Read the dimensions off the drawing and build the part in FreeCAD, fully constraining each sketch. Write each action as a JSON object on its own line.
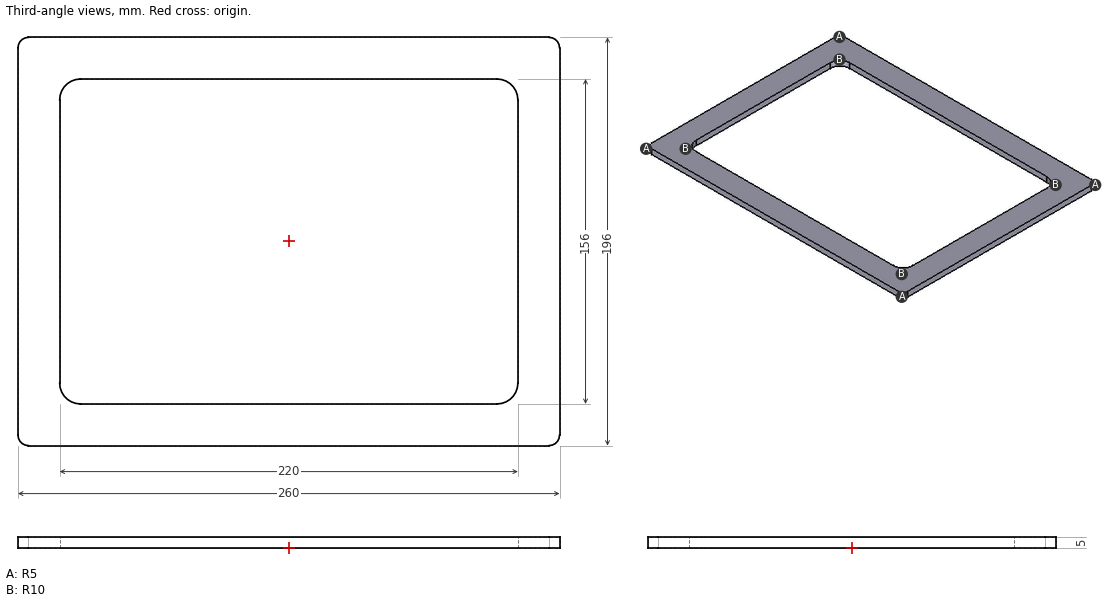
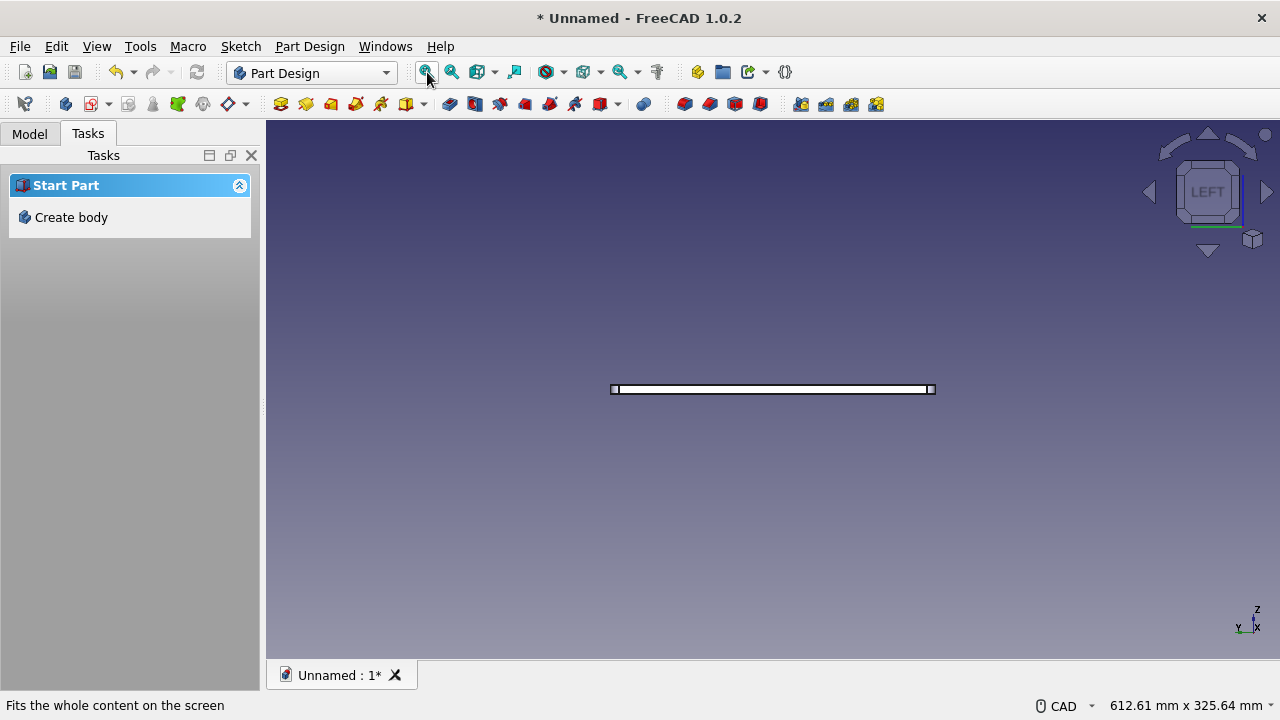
{"action": "key", "text": "v 3"}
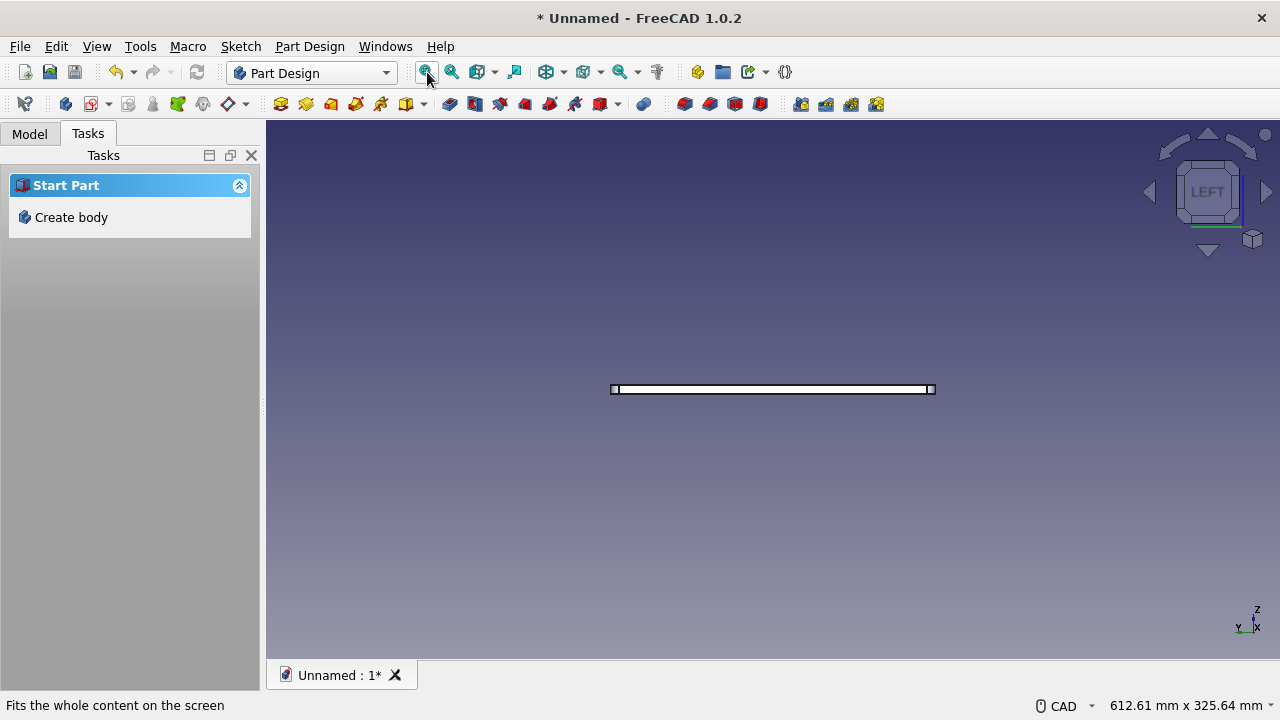
{"action": "key", "text": "0"}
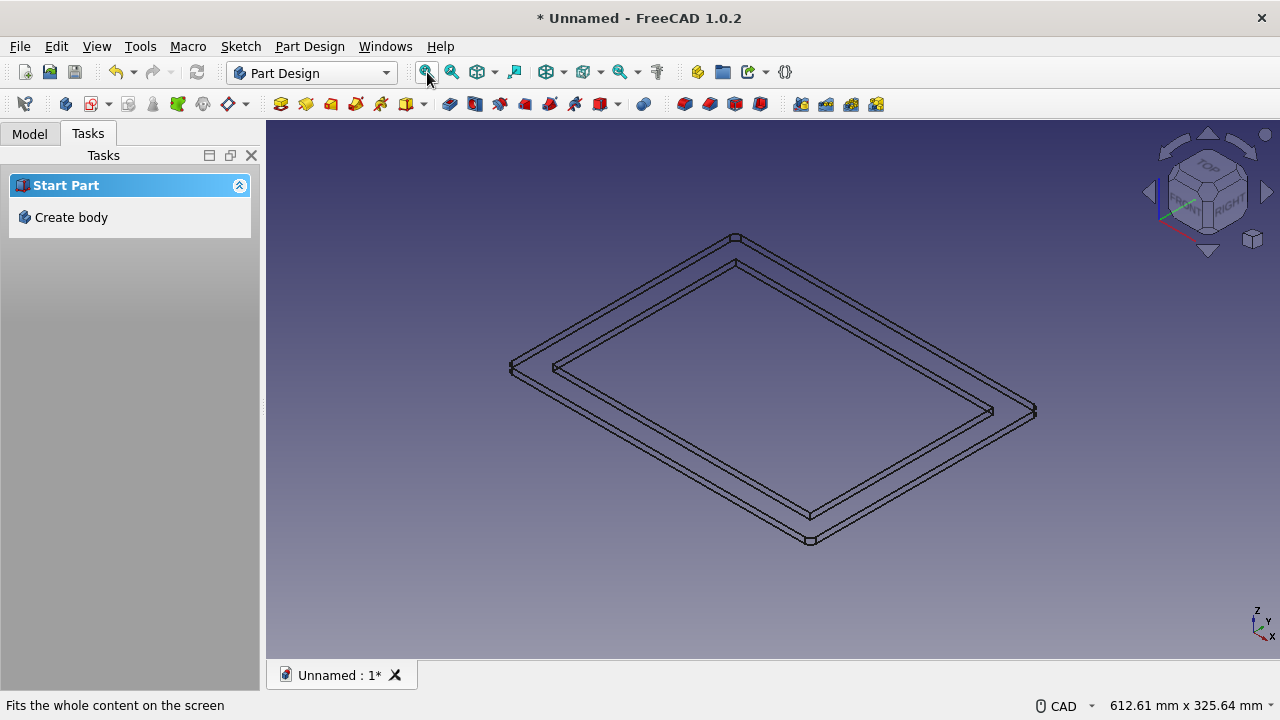
{"action": "scroll", "coordinate": [736, 261], "scroll_direction": "up", "scroll_amount": 8}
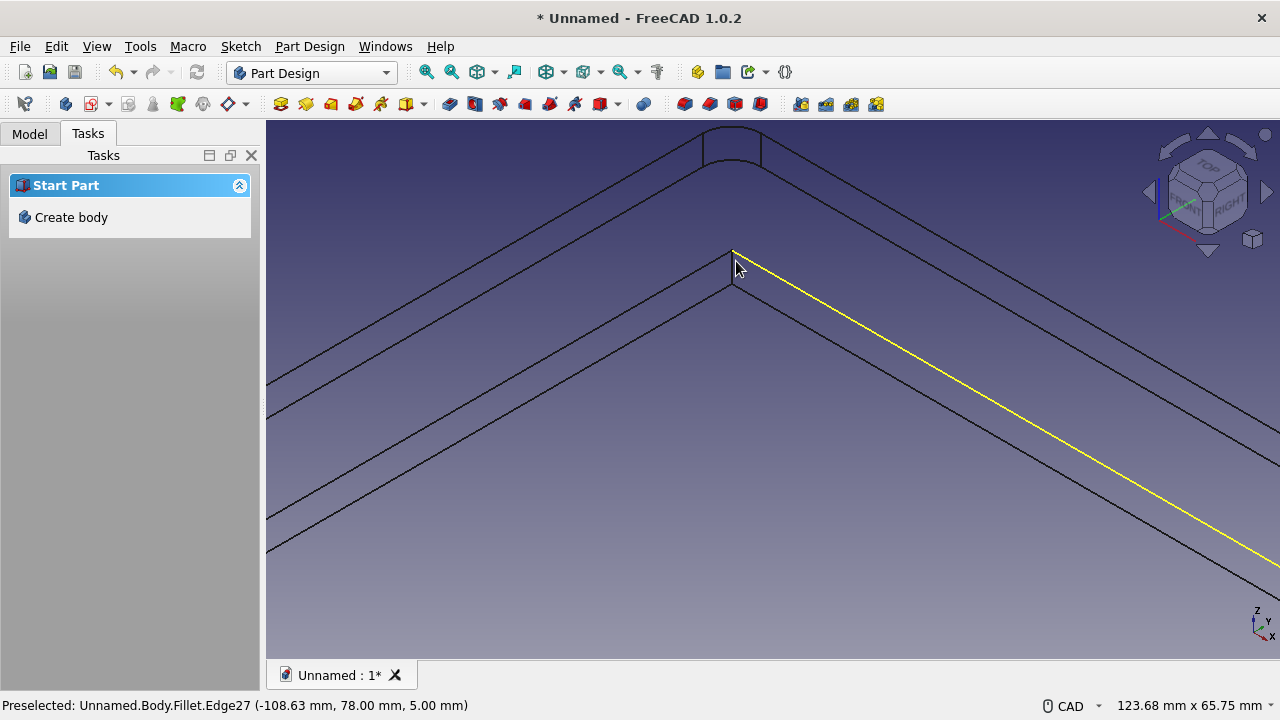
{"action": "left_click", "coordinate": [732, 266]}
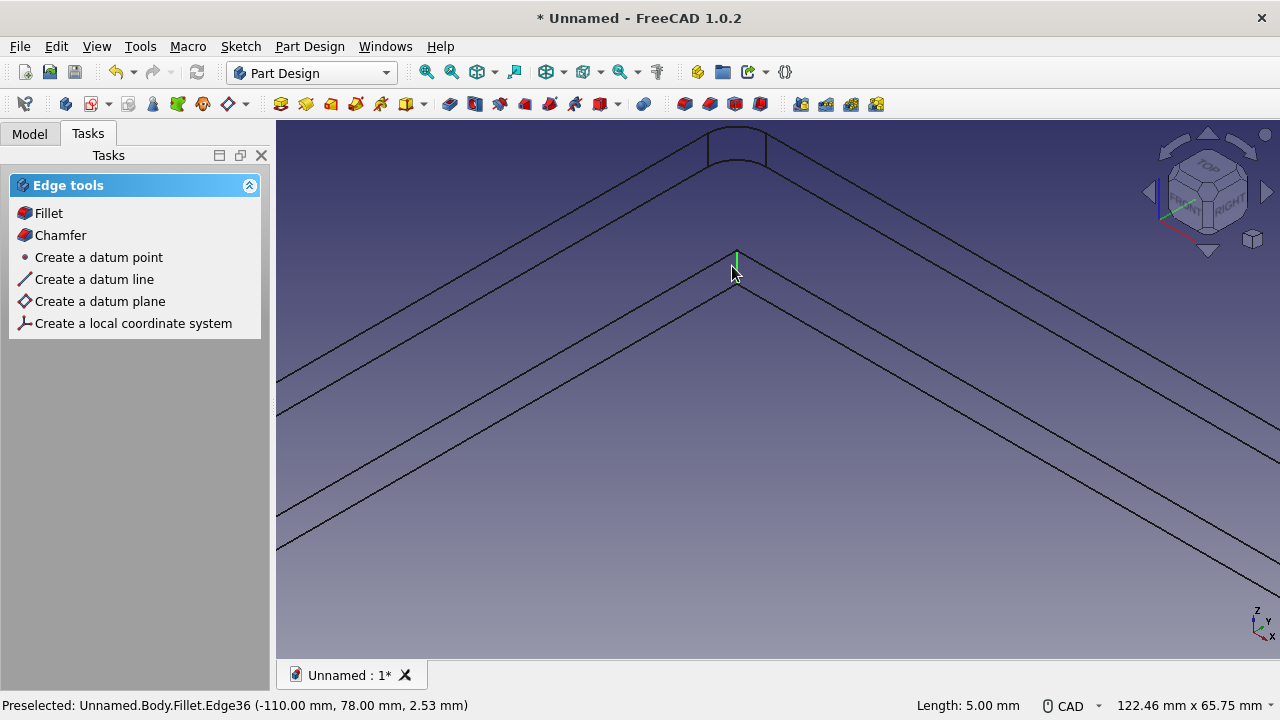
{"action": "left_click", "coordinate": [427, 72]}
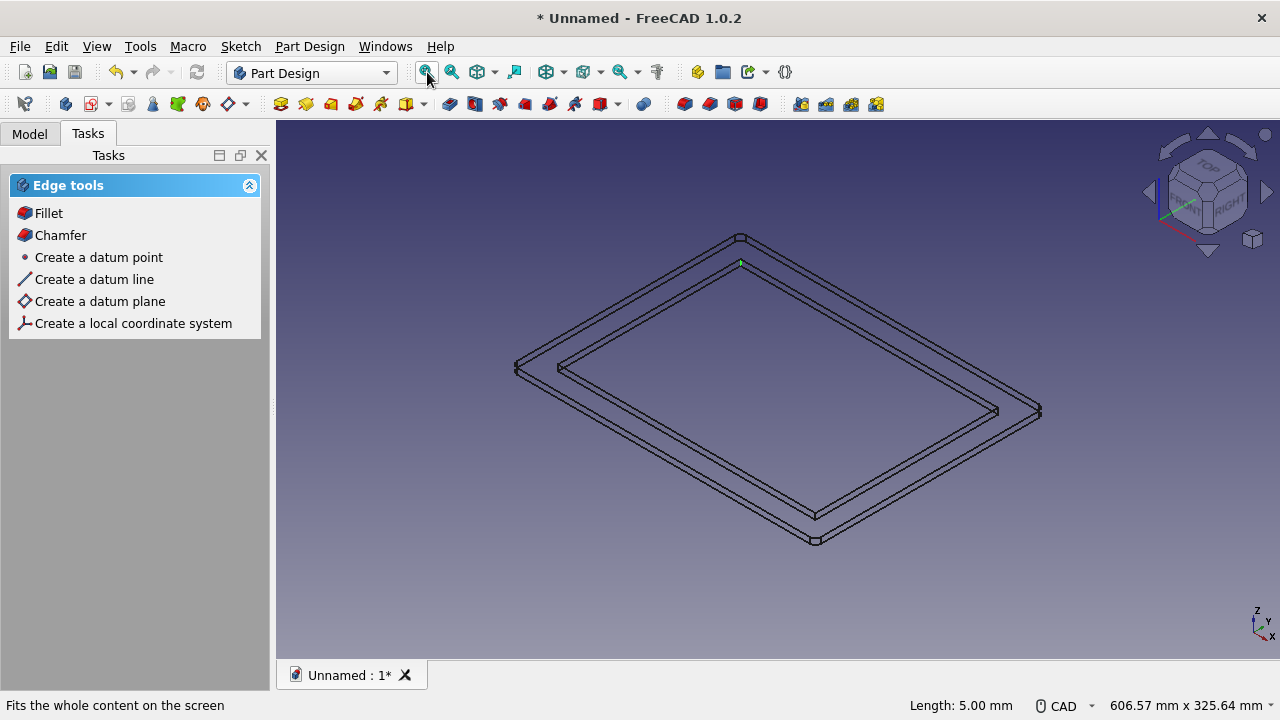
{"action": "key", "text": "2"}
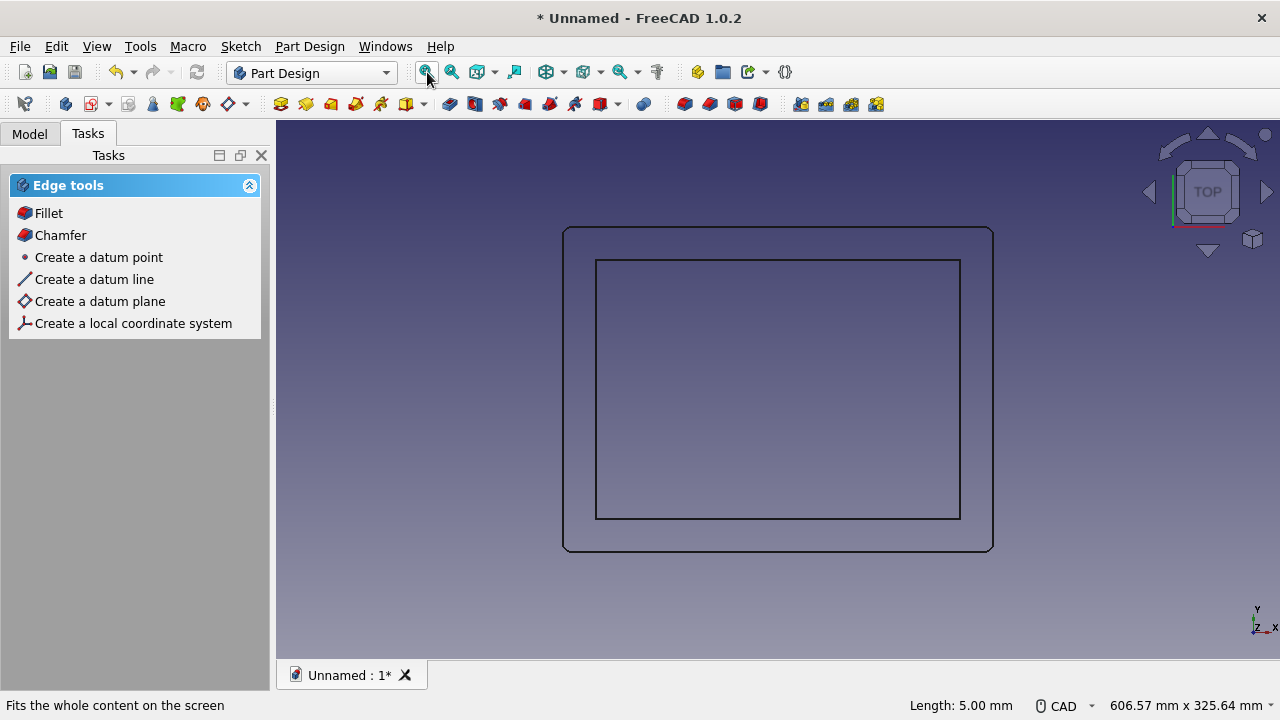
{"action": "scroll", "coordinate": [596, 518], "scroll_direction": "up", "scroll_amount": 8}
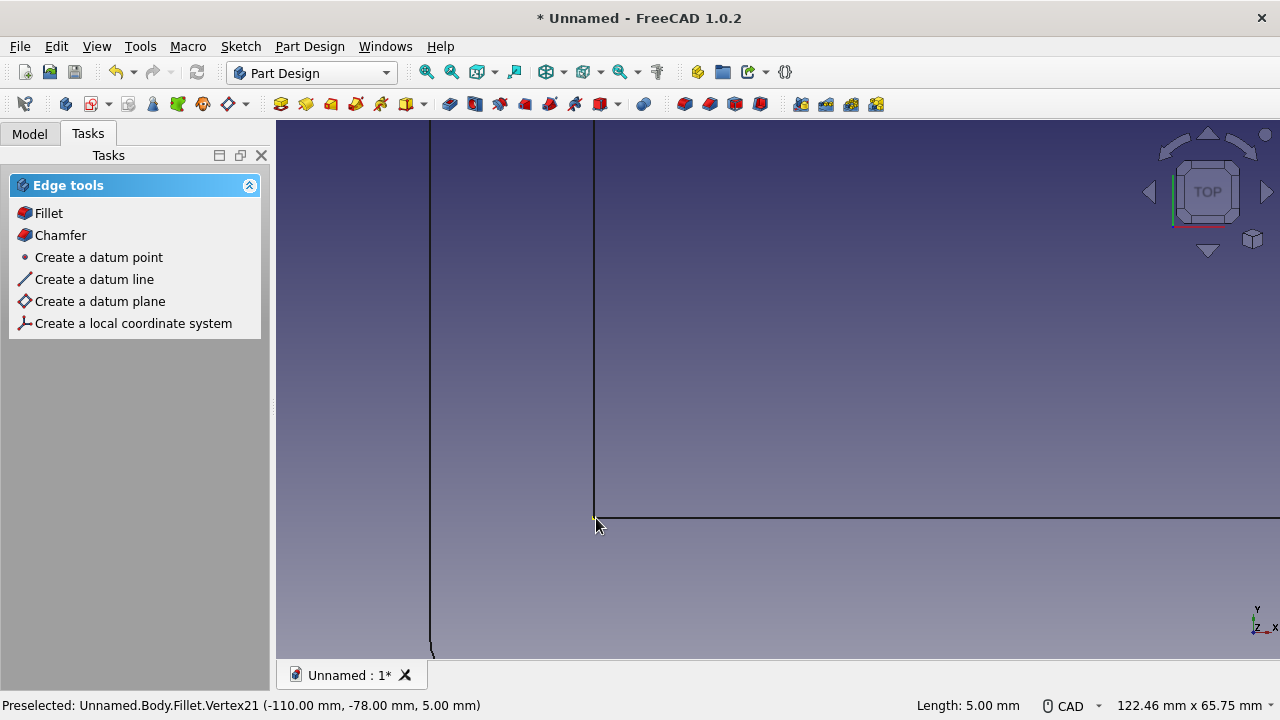
{"action": "left_click", "coordinate": [427, 72]}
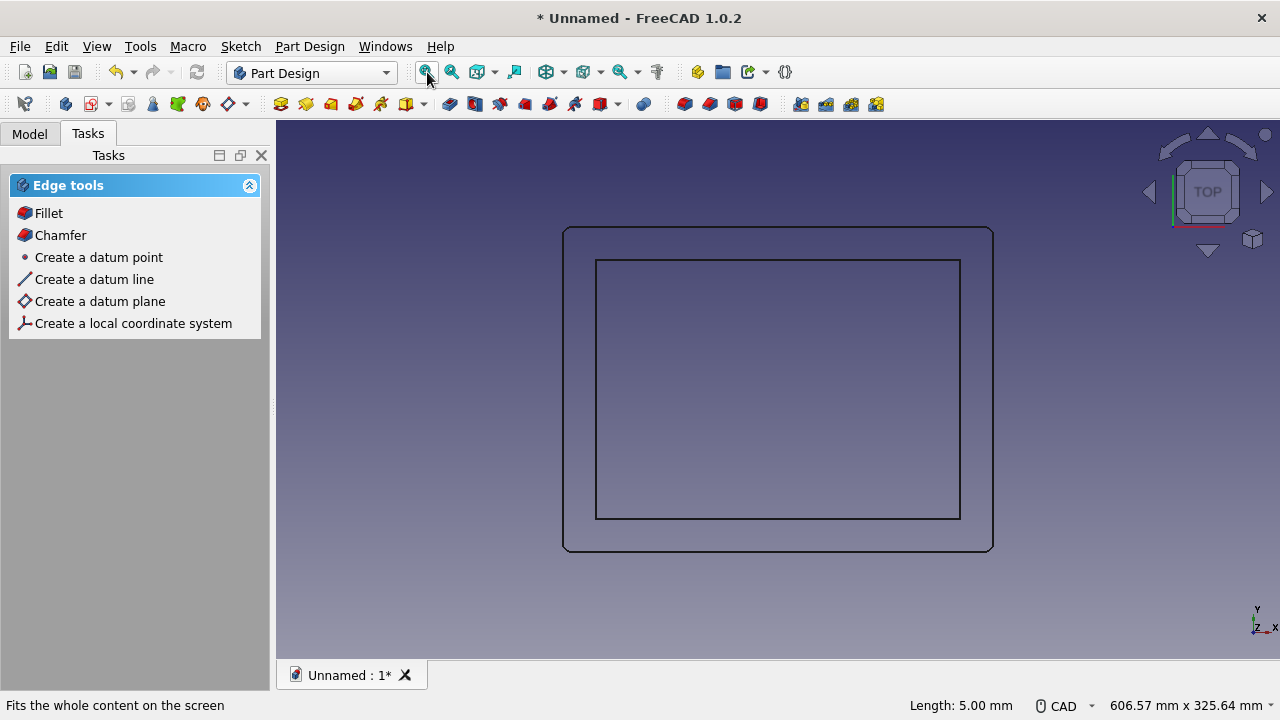
{"action": "key", "text": "1"}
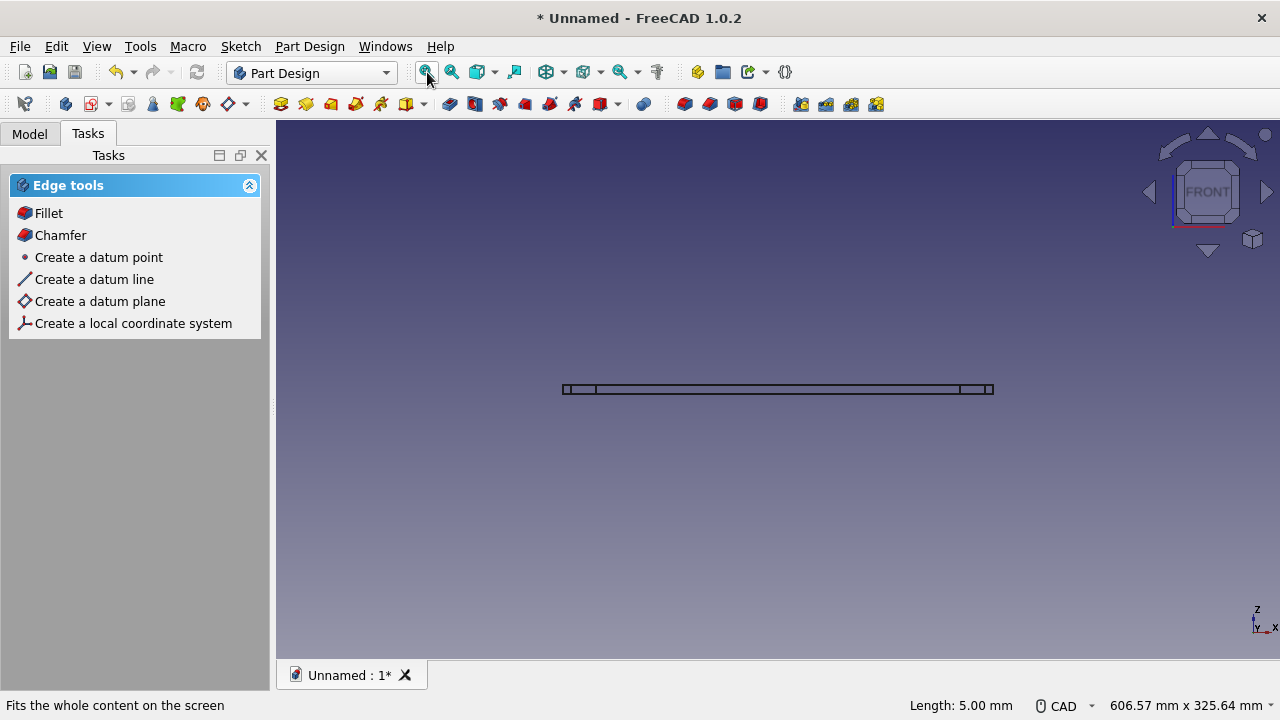
{"action": "key", "text": "v f"}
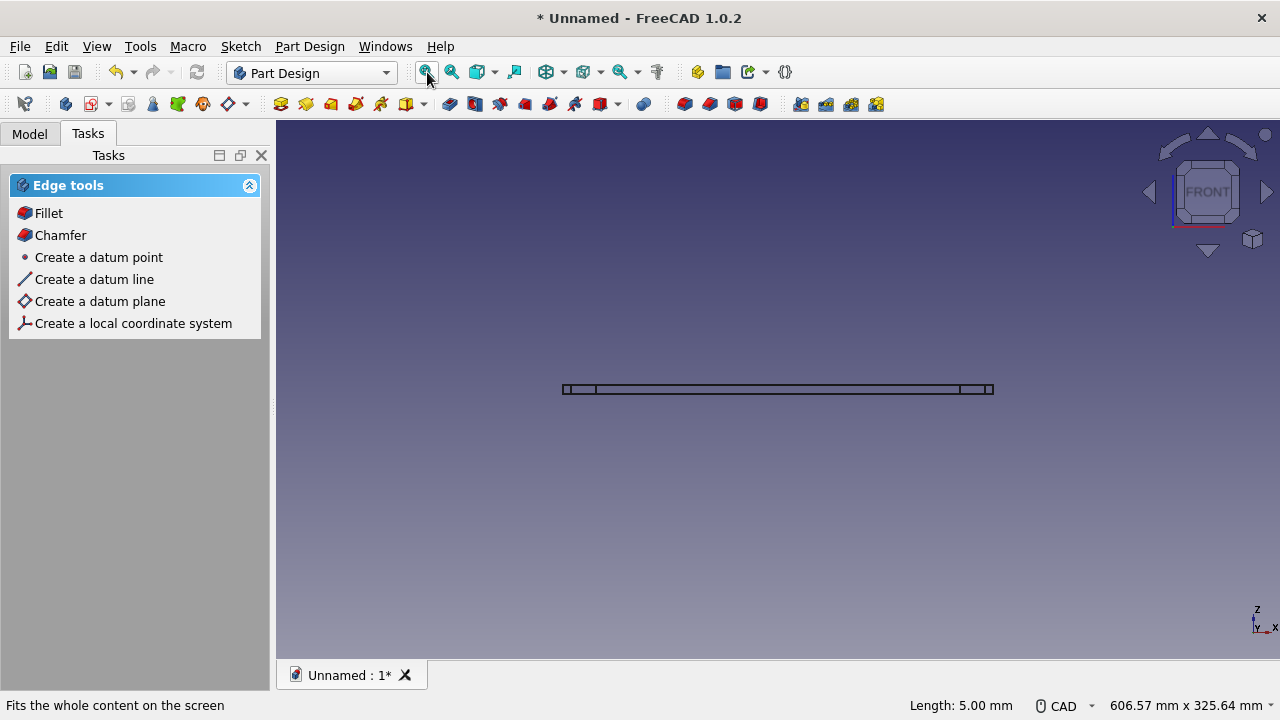
{"action": "scroll", "coordinate": [596, 389], "scroll_direction": "up", "scroll_amount": 8}